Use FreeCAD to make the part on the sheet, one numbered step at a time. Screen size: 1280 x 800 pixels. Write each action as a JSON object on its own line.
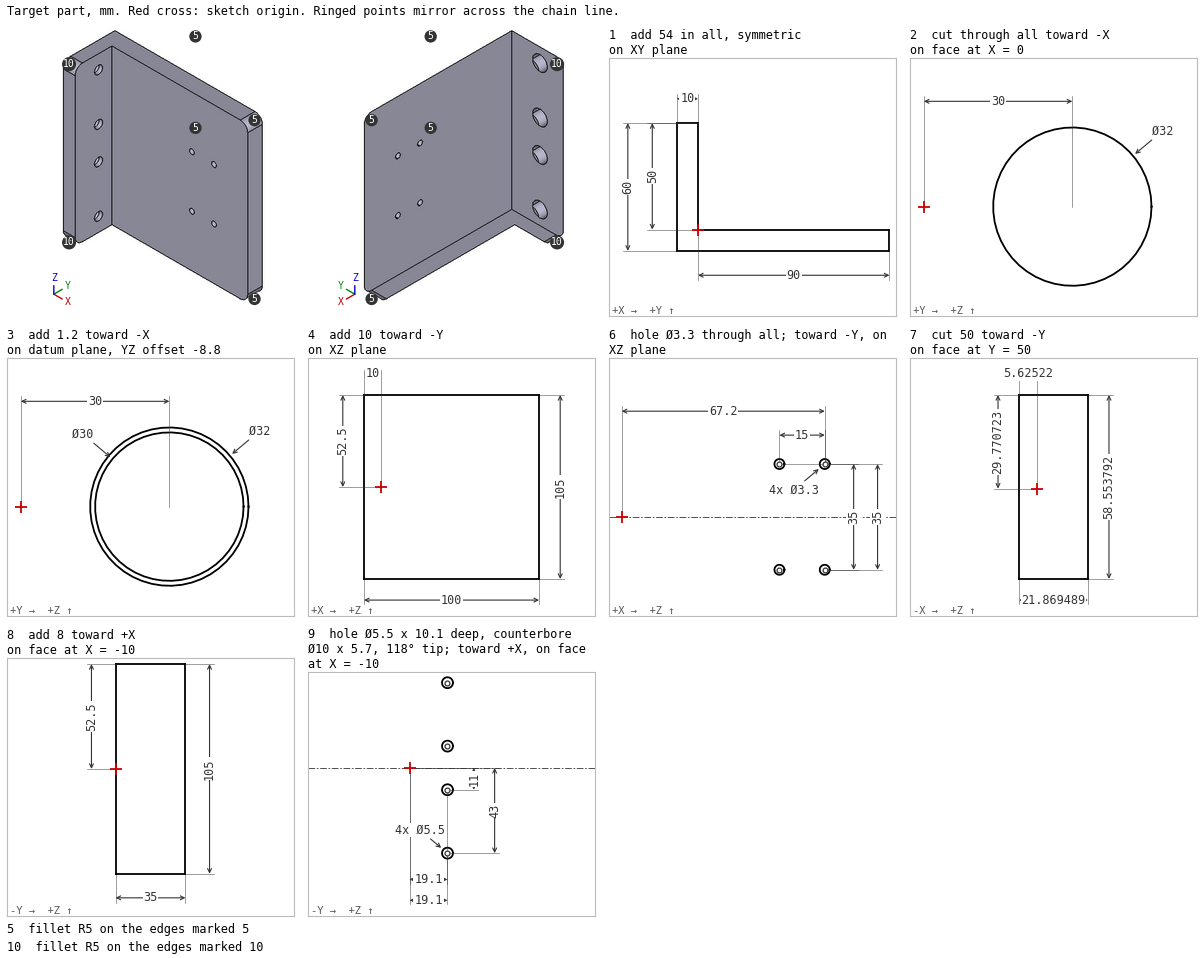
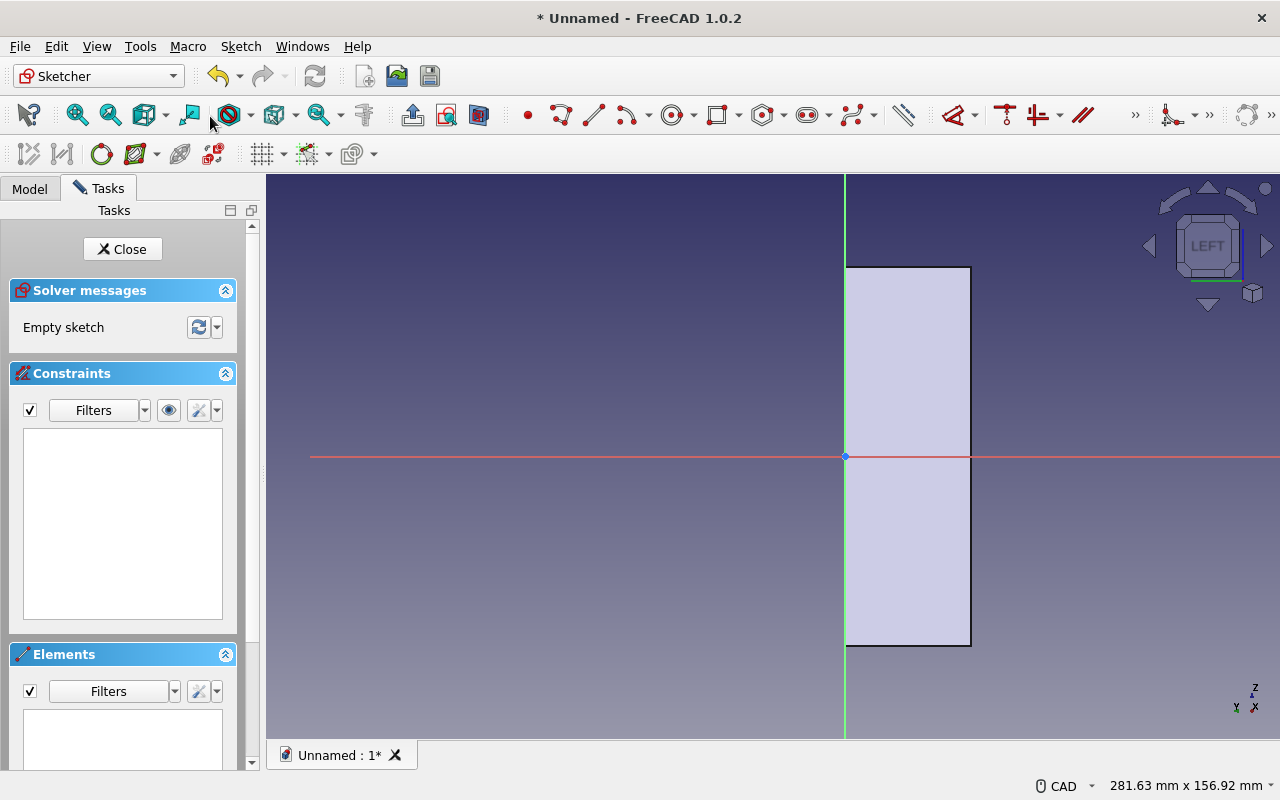
{"action": "left_click", "coordinate": [672, 116]}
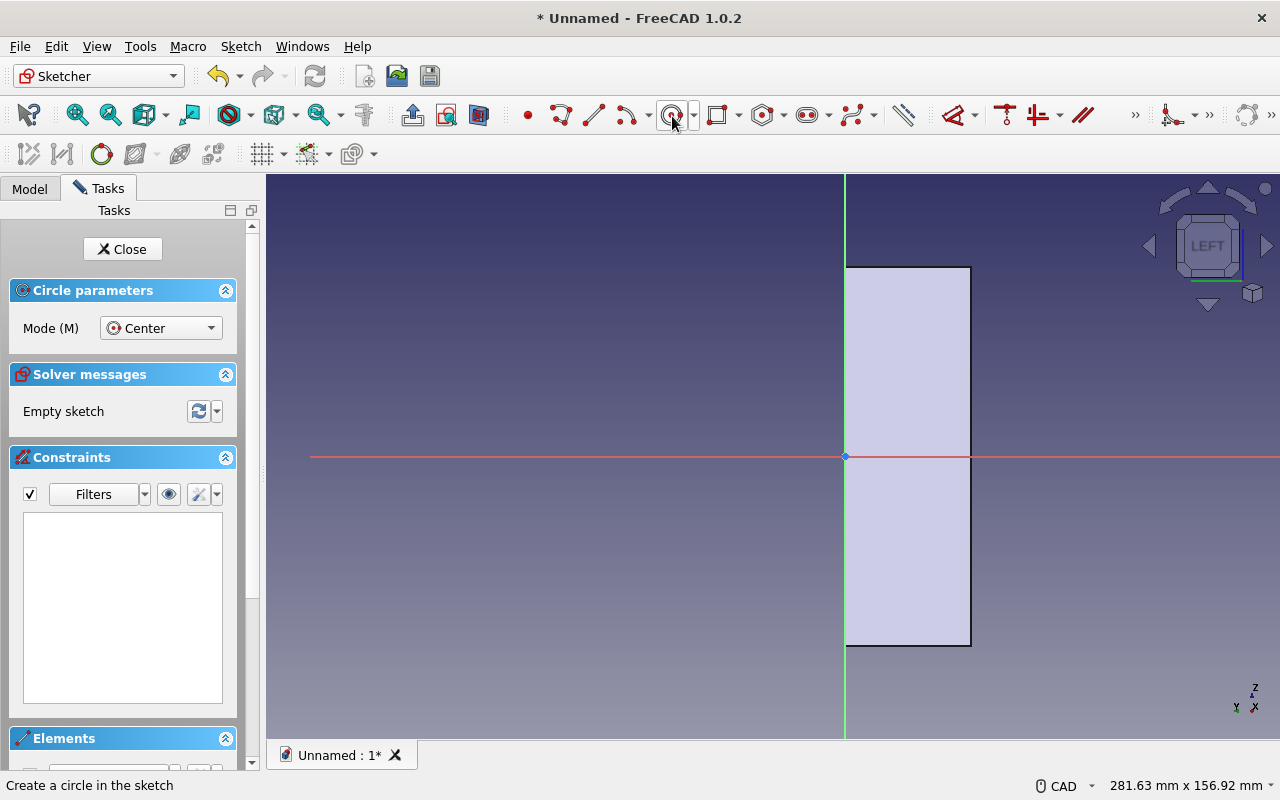
{"action": "scroll", "coordinate": [914, 611], "scroll_direction": "up", "scroll_amount": 5}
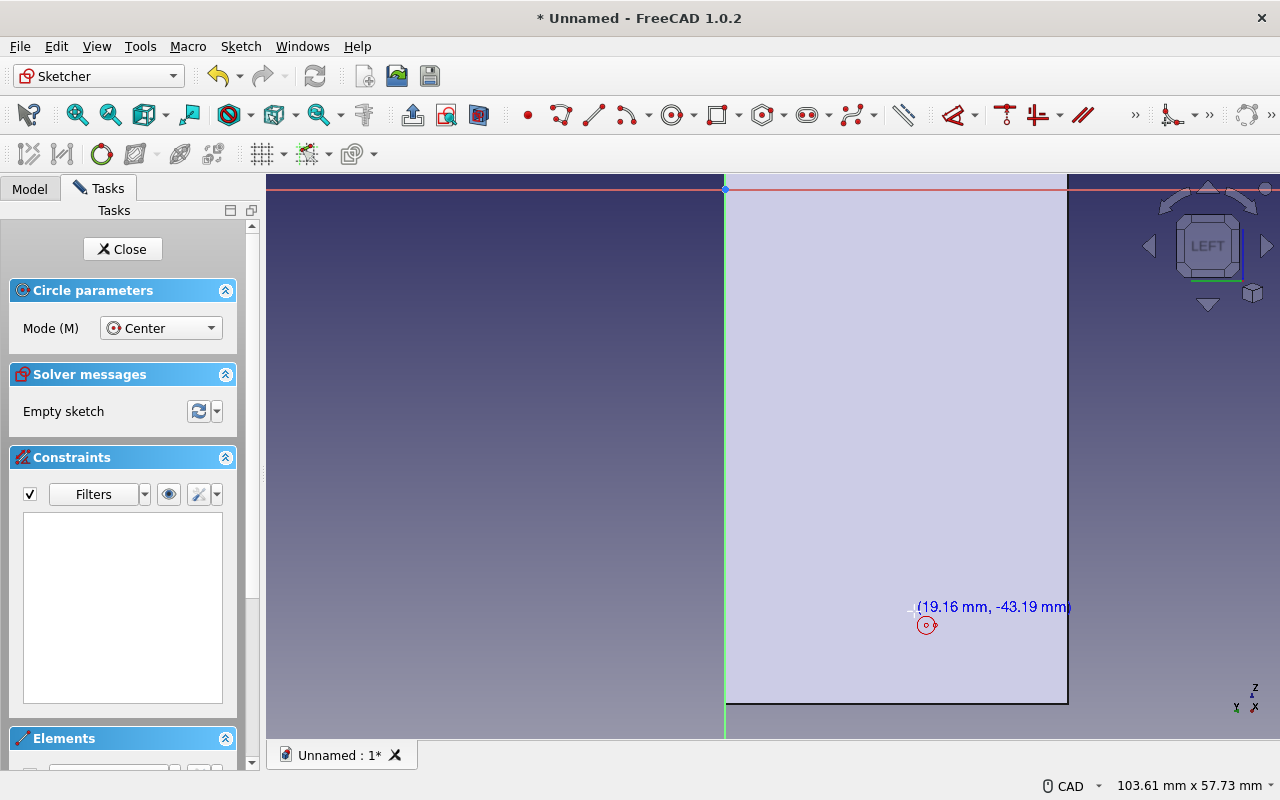
{"action": "left_click", "coordinate": [912, 611]}
{"action": "mouse_move", "coordinate": [931, 592]}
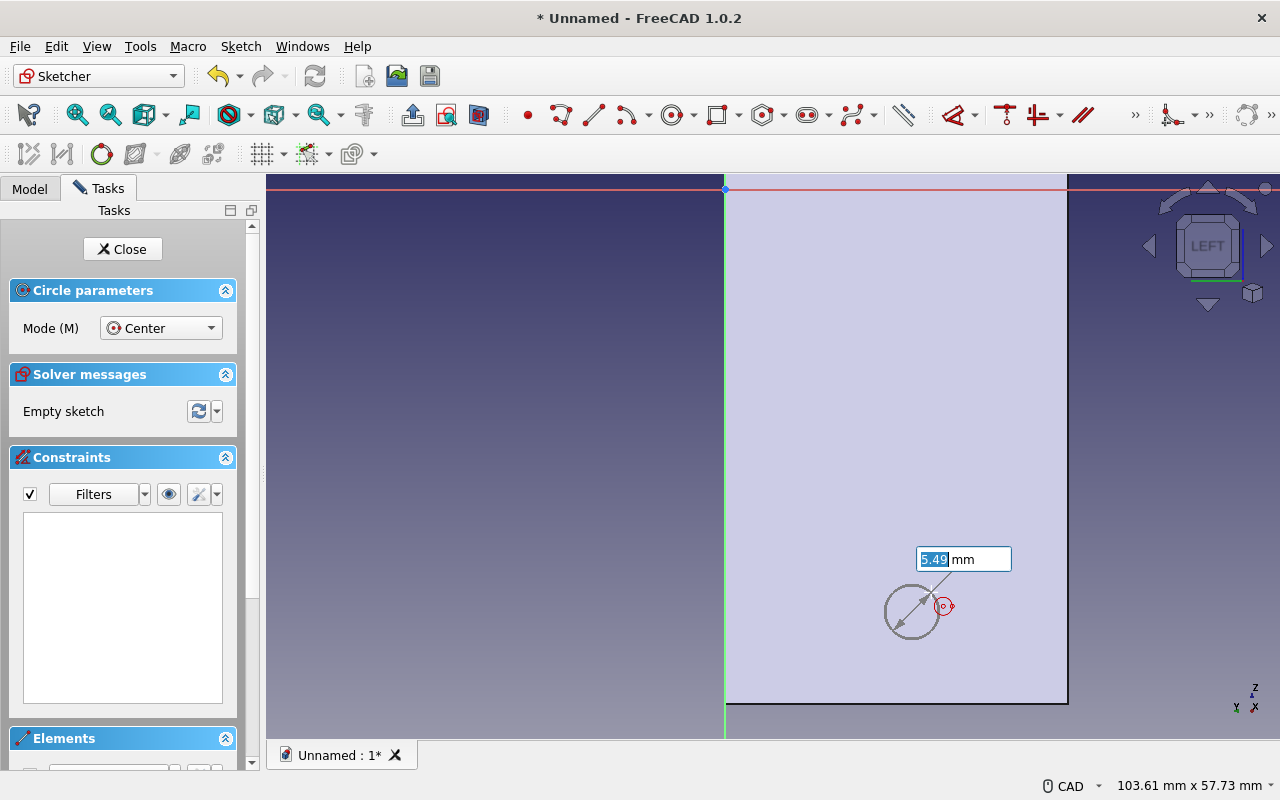
{"action": "type", "text": "5.5"}
{"action": "key", "text": "Return"}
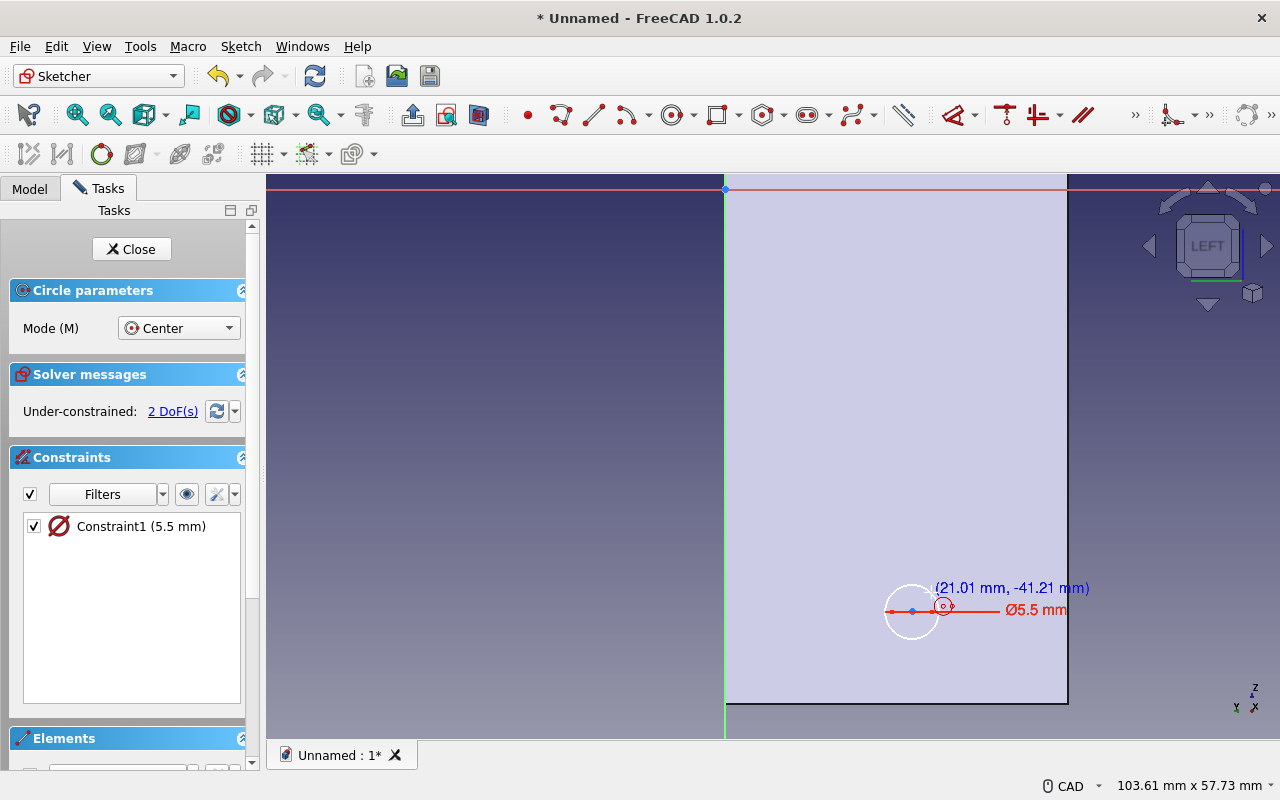
{"action": "left_click", "coordinate": [912, 297]}
{"action": "mouse_move", "coordinate": [931, 278]}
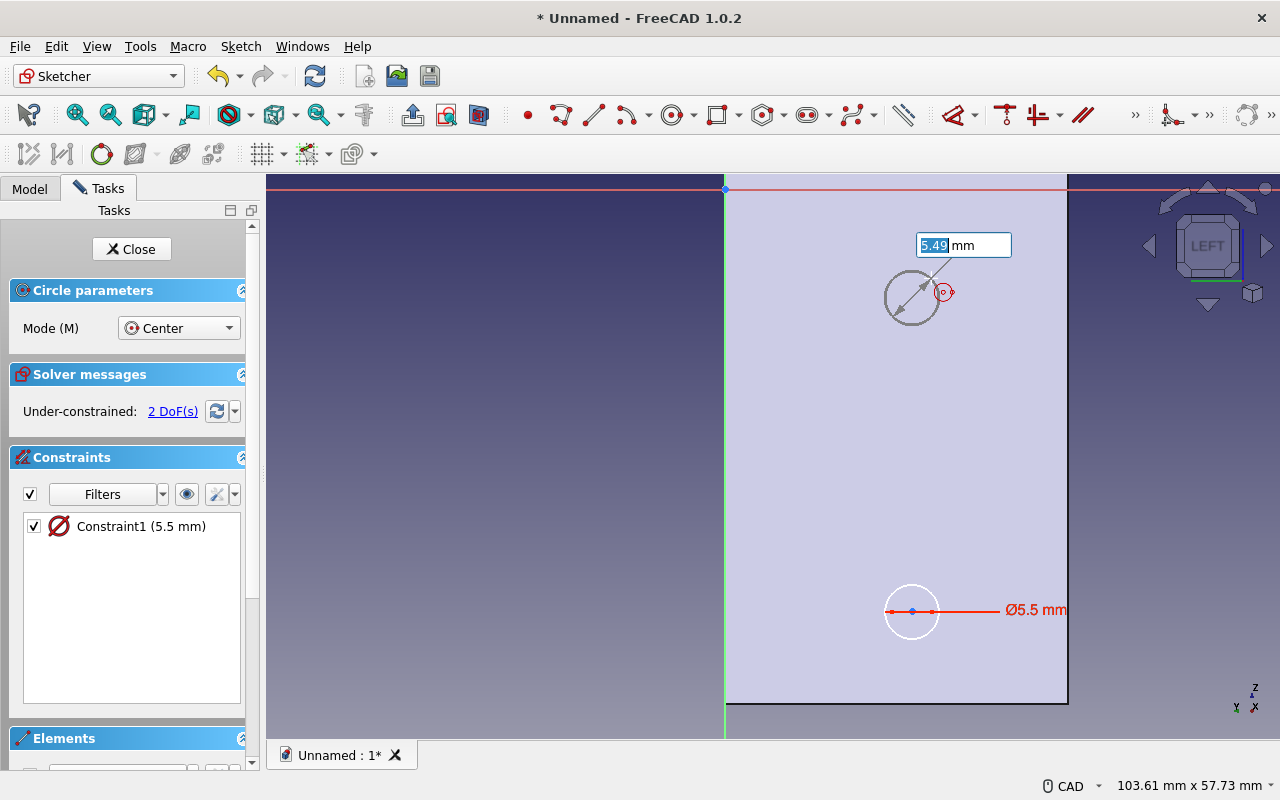
{"action": "type", "text": "5.5"}
{"action": "key", "text": "Return"}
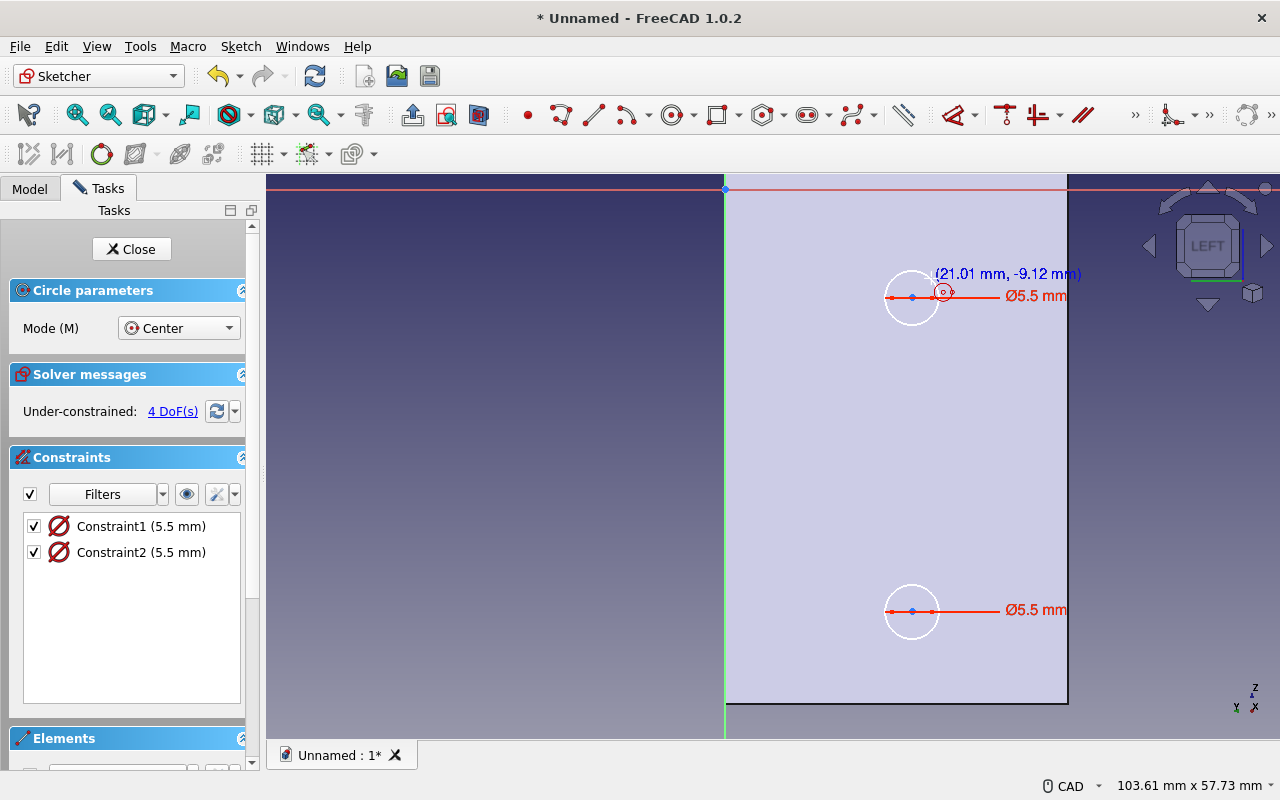
{"action": "scroll", "coordinate": [630, 612], "scroll_direction": "down", "scroll_amount": 5}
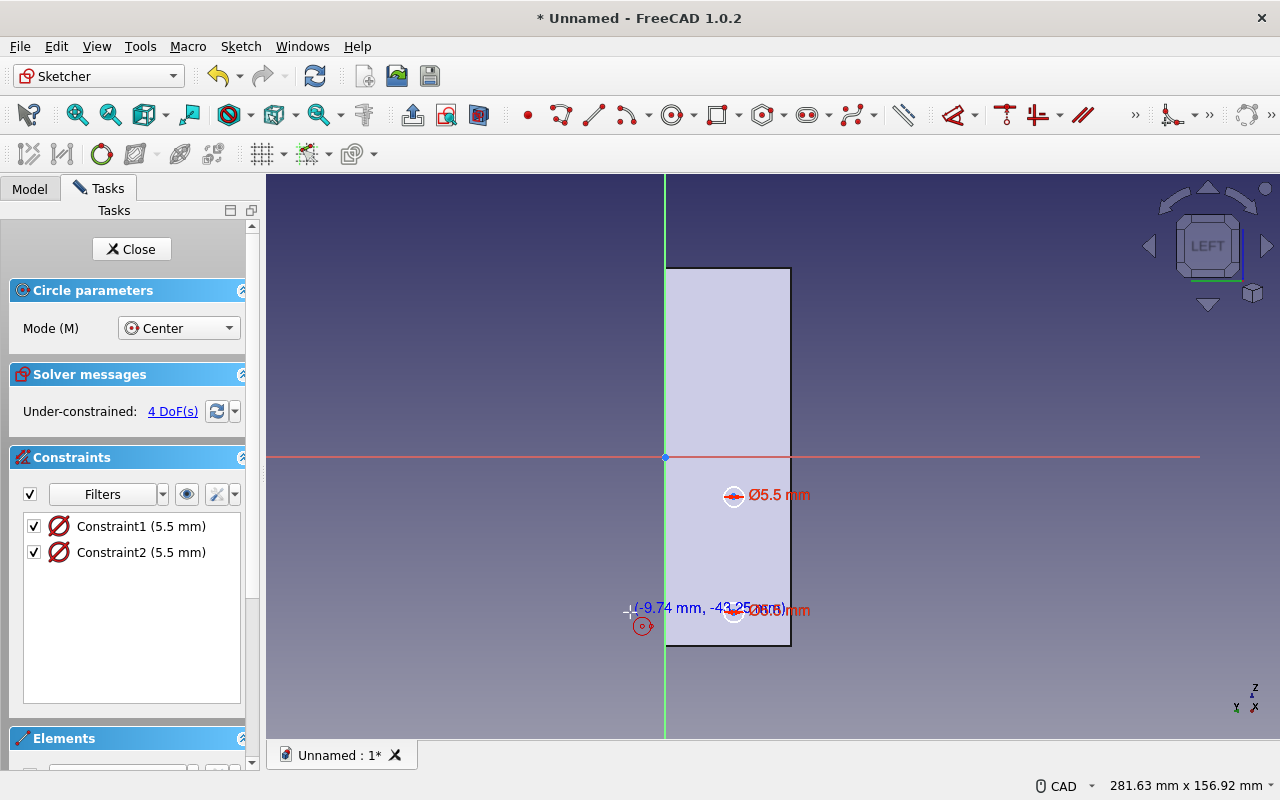
{"action": "scroll", "coordinate": [734, 418], "scroll_direction": "up", "scroll_amount": 5}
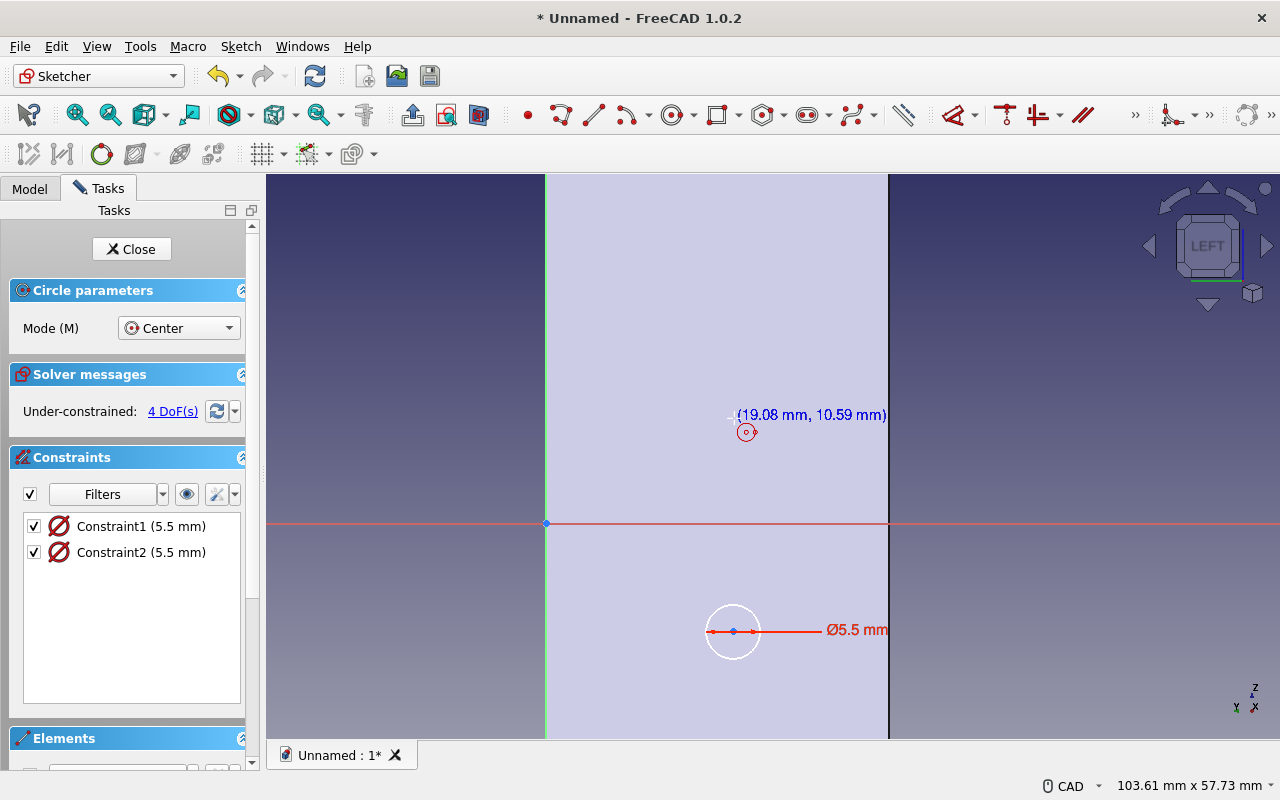
{"action": "left_click", "coordinate": [733, 416]}
{"action": "mouse_move", "coordinate": [752, 397]}